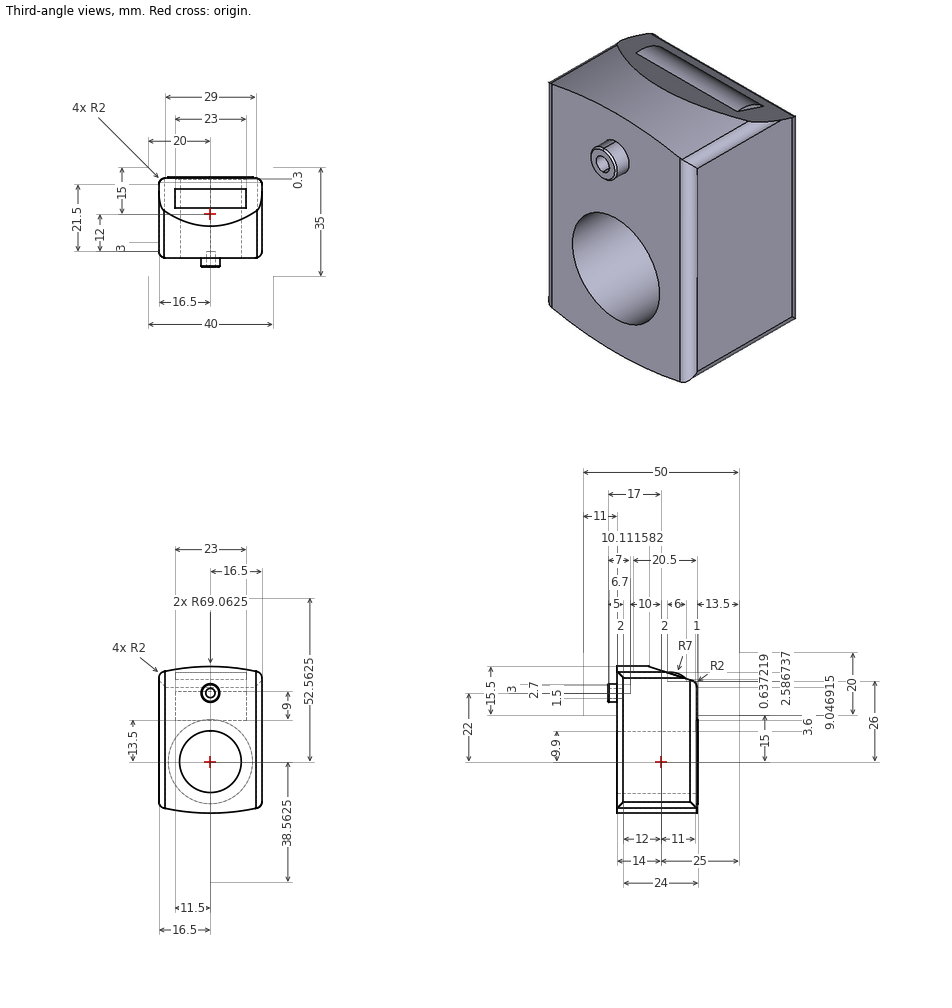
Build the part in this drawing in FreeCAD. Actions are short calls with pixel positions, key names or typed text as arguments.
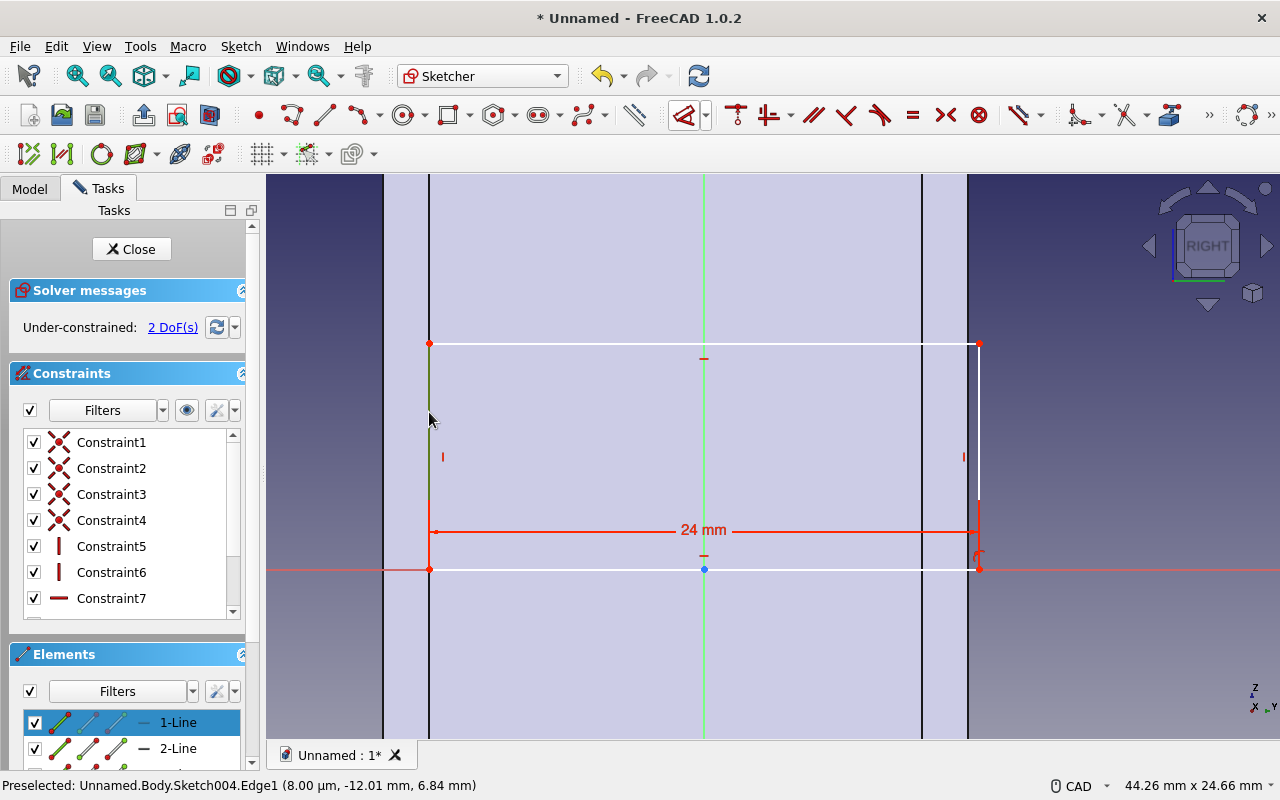
click(706, 116)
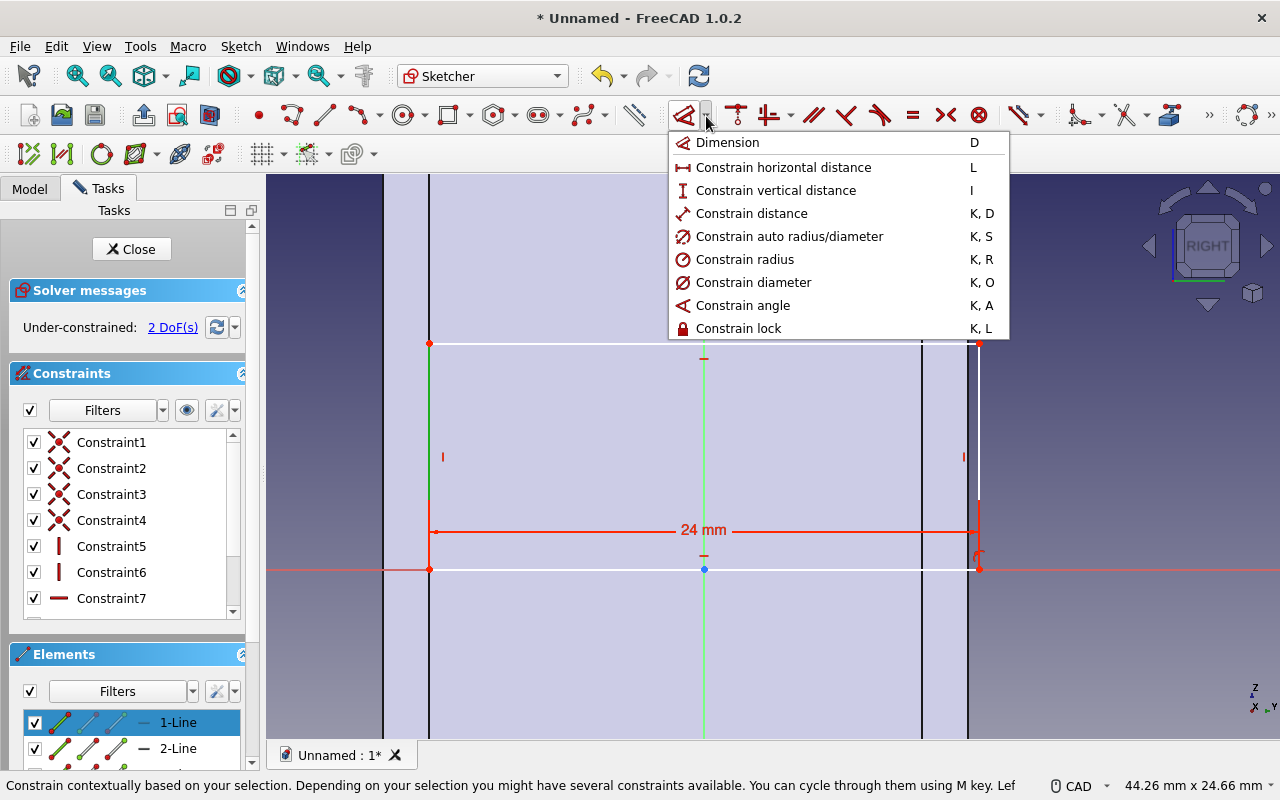
click(839, 190)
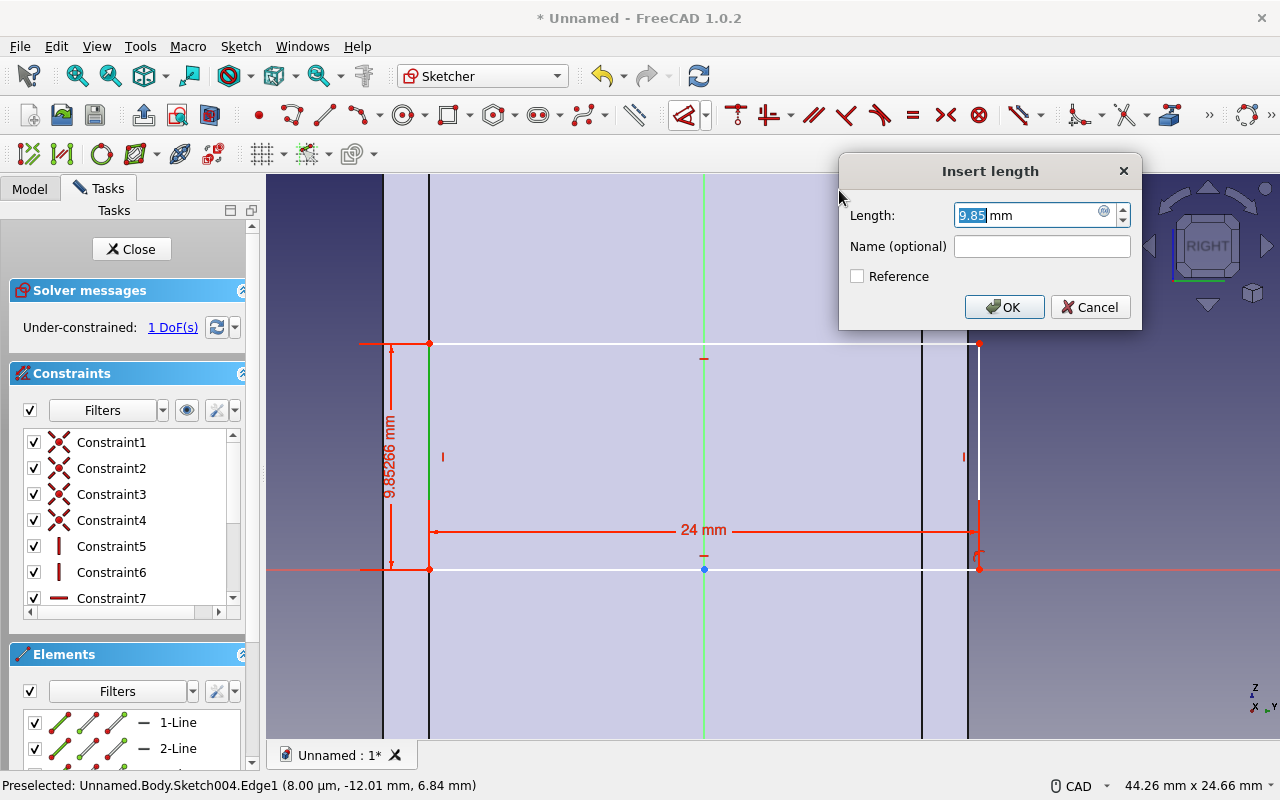
text(9.9)
key(Return)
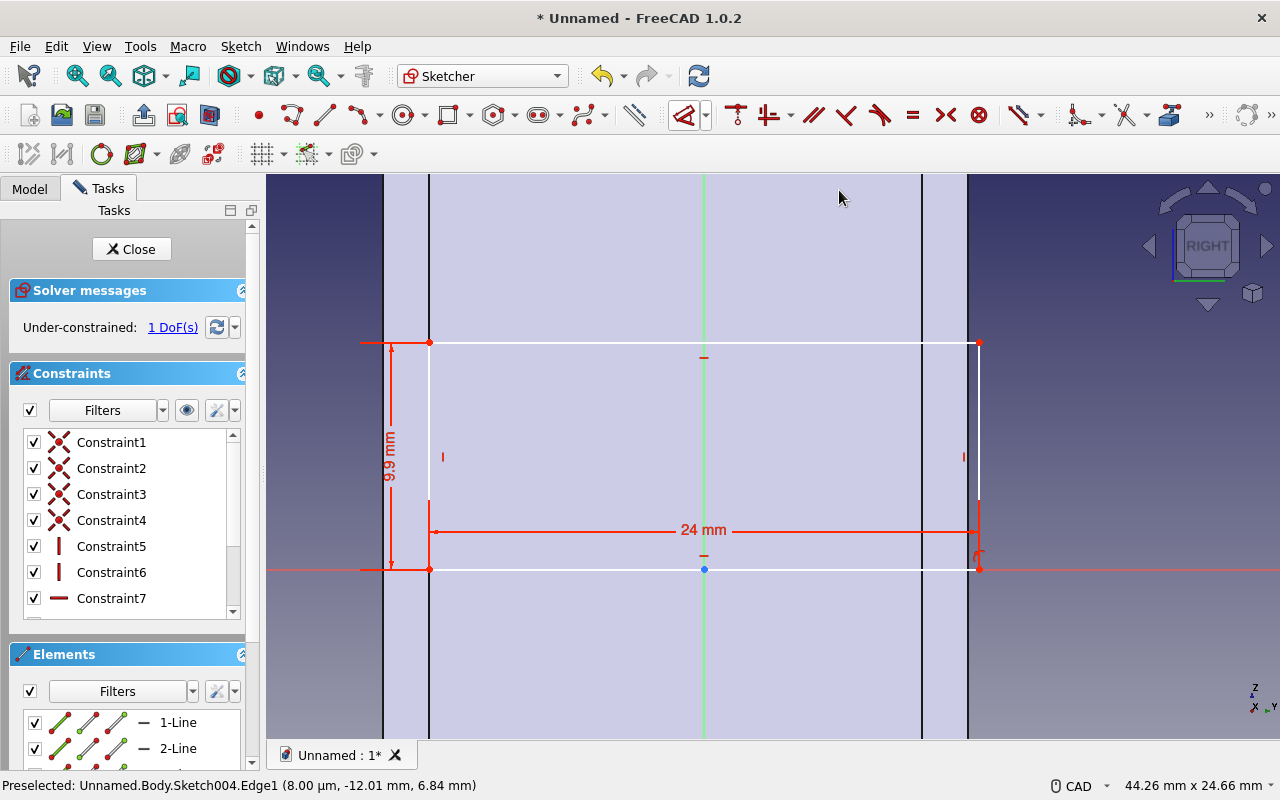
click(429, 343)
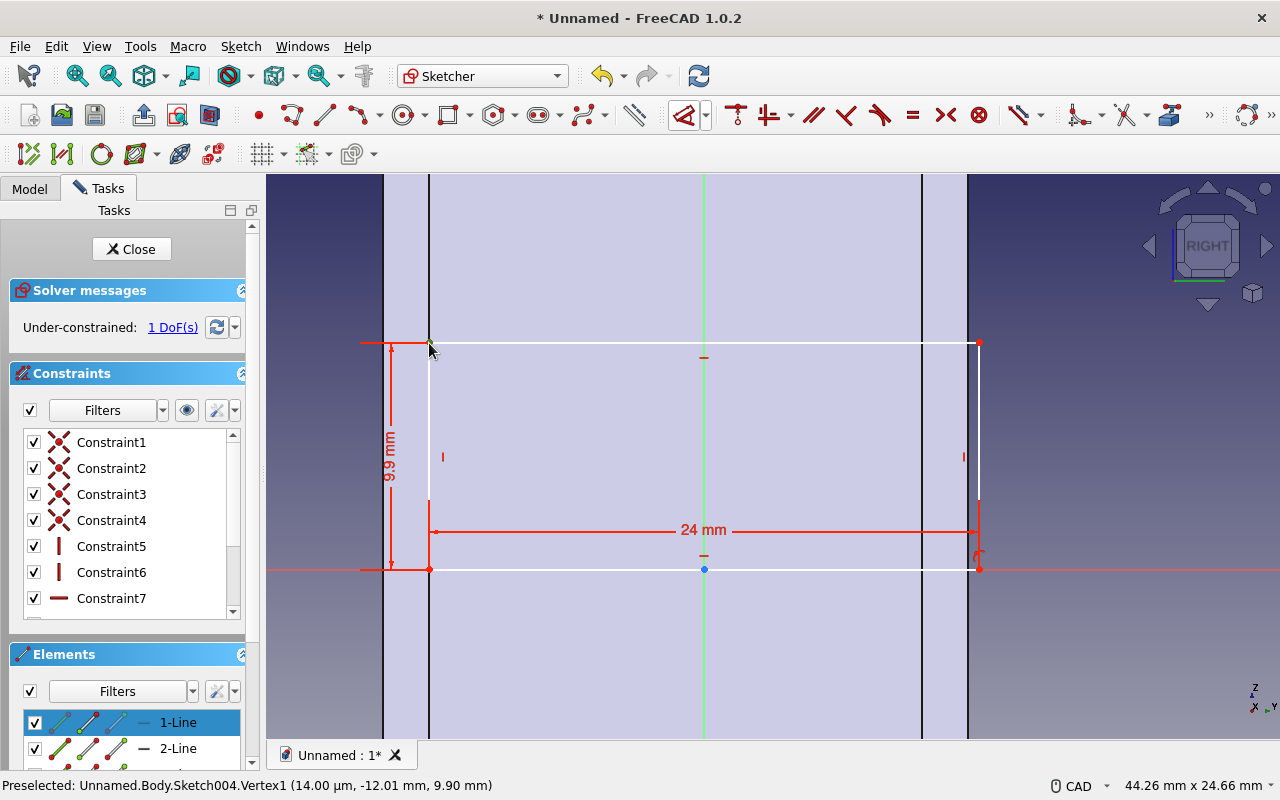
click(706, 116)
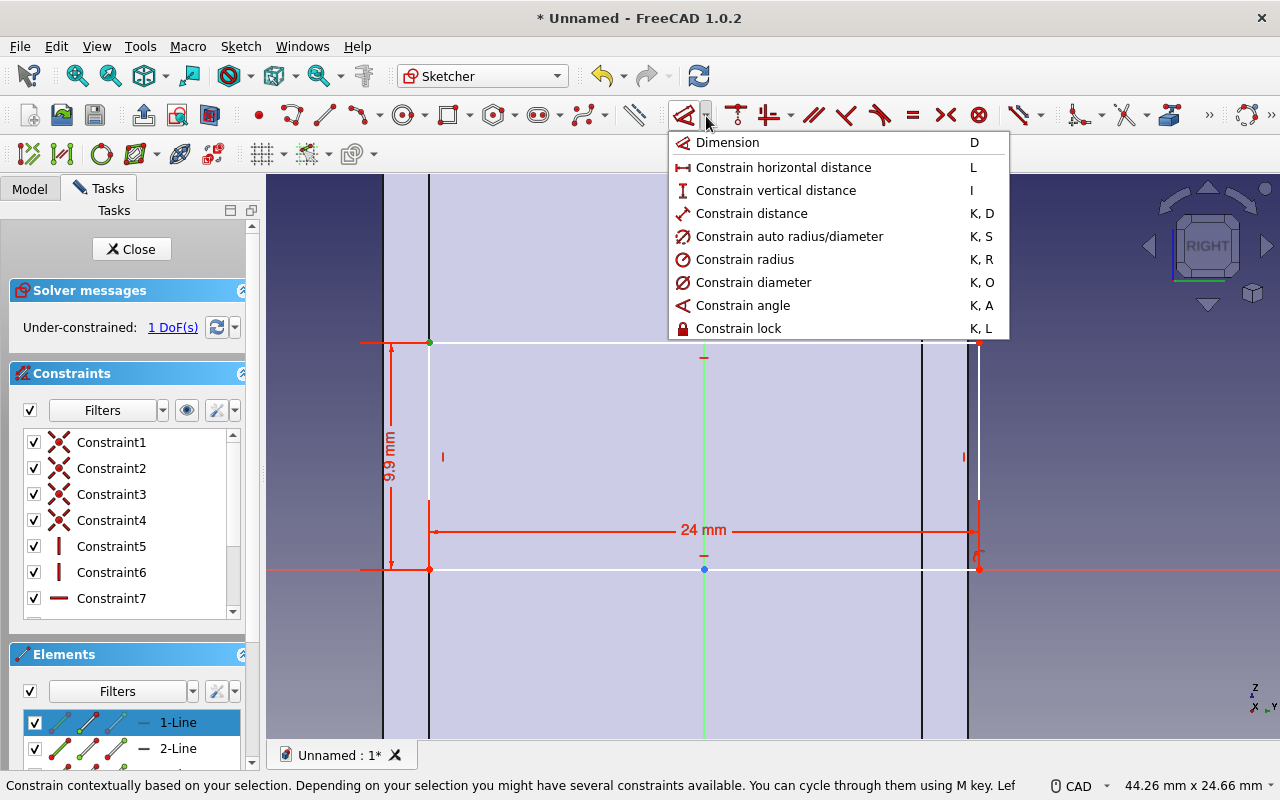
click(839, 168)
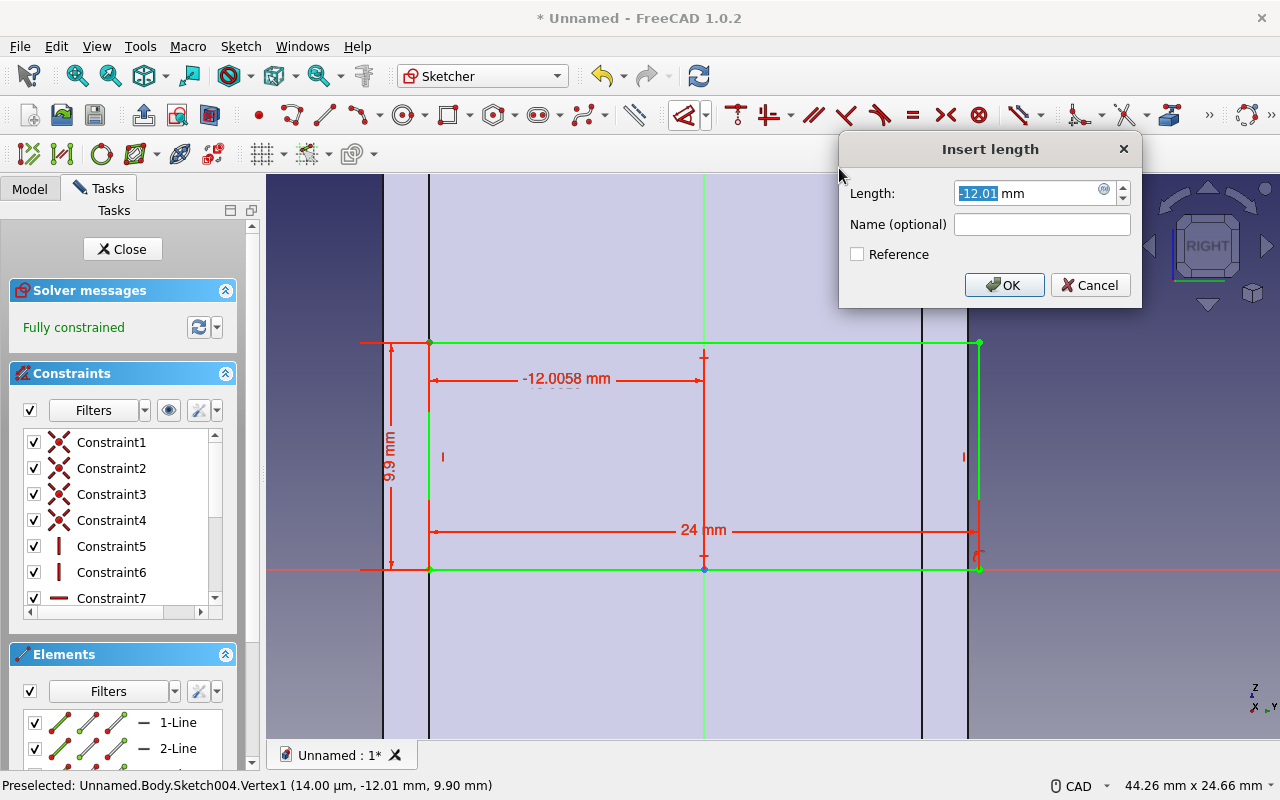
text(-12)
key(Return)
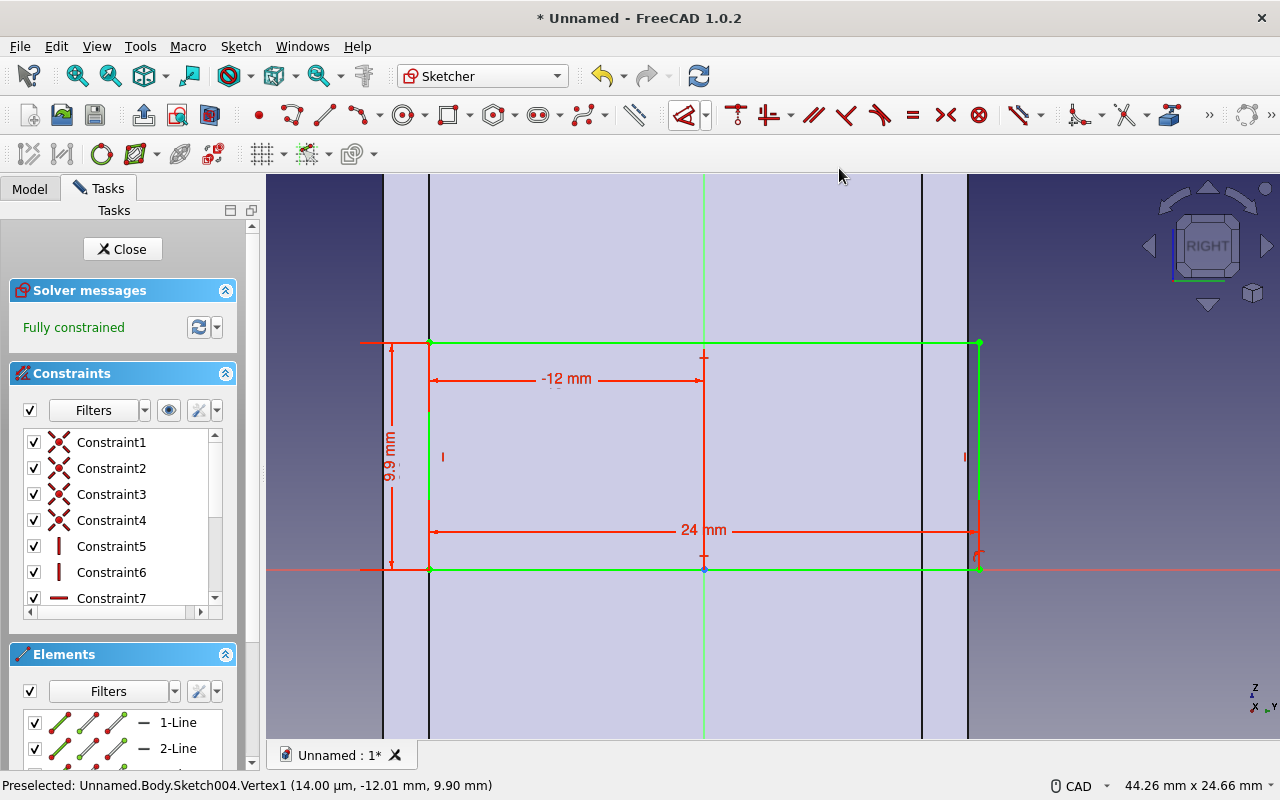
click(123, 249)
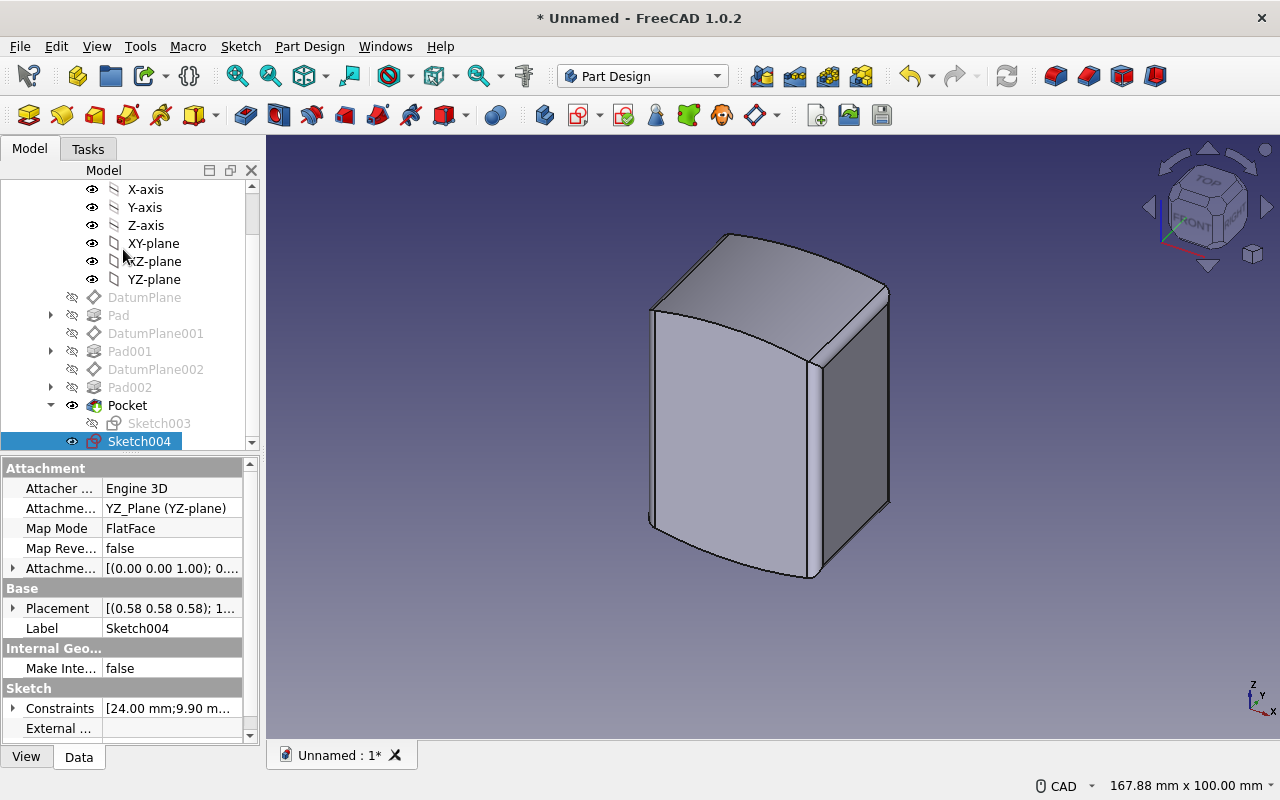
click(312, 116)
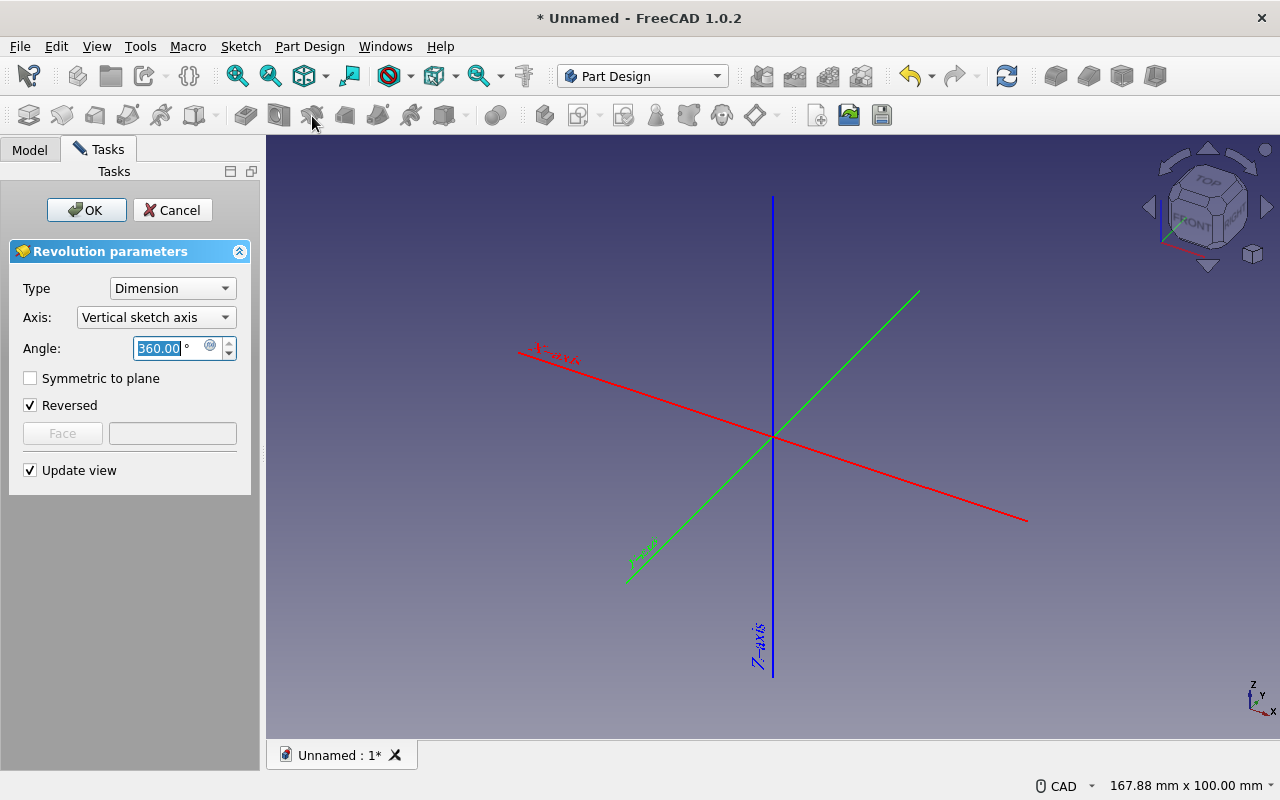
click(157, 318)